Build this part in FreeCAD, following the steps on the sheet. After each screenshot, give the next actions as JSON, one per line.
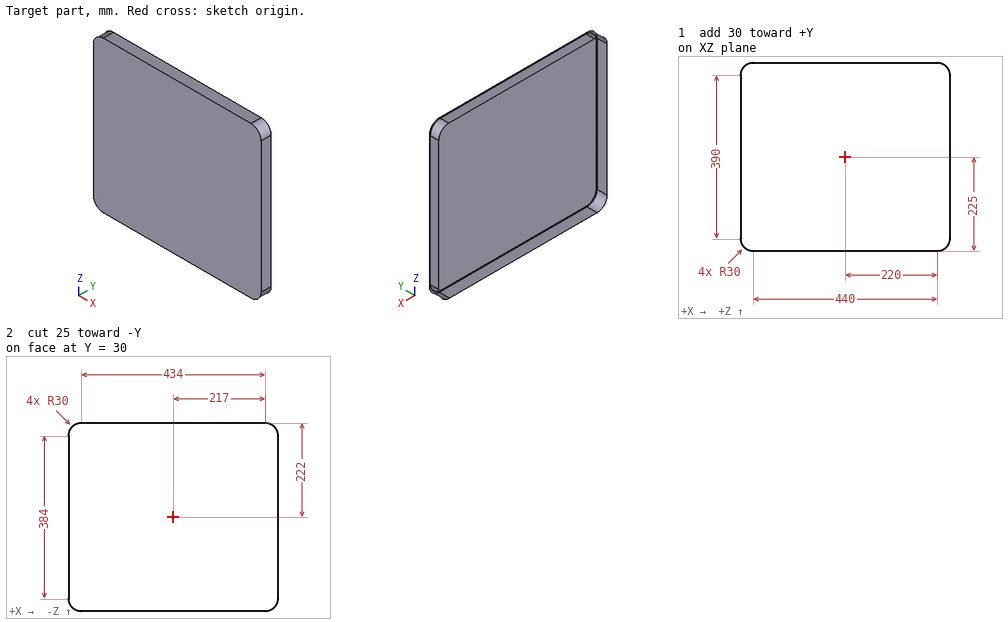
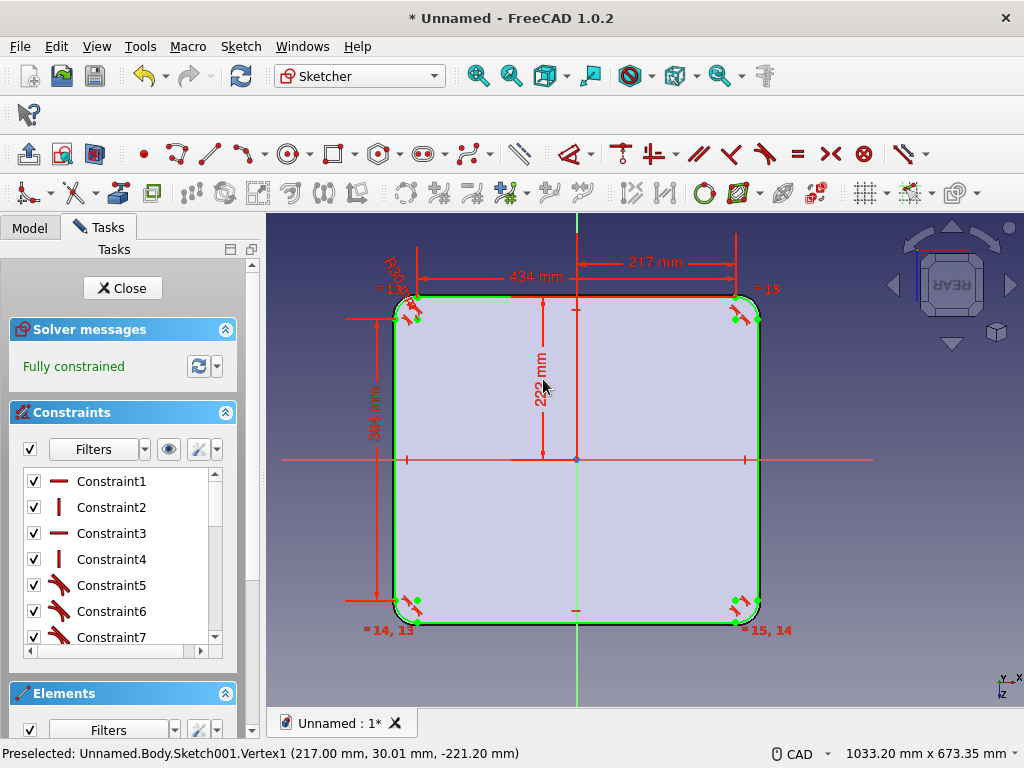
{"action": "left_click", "coordinate": [123, 288]}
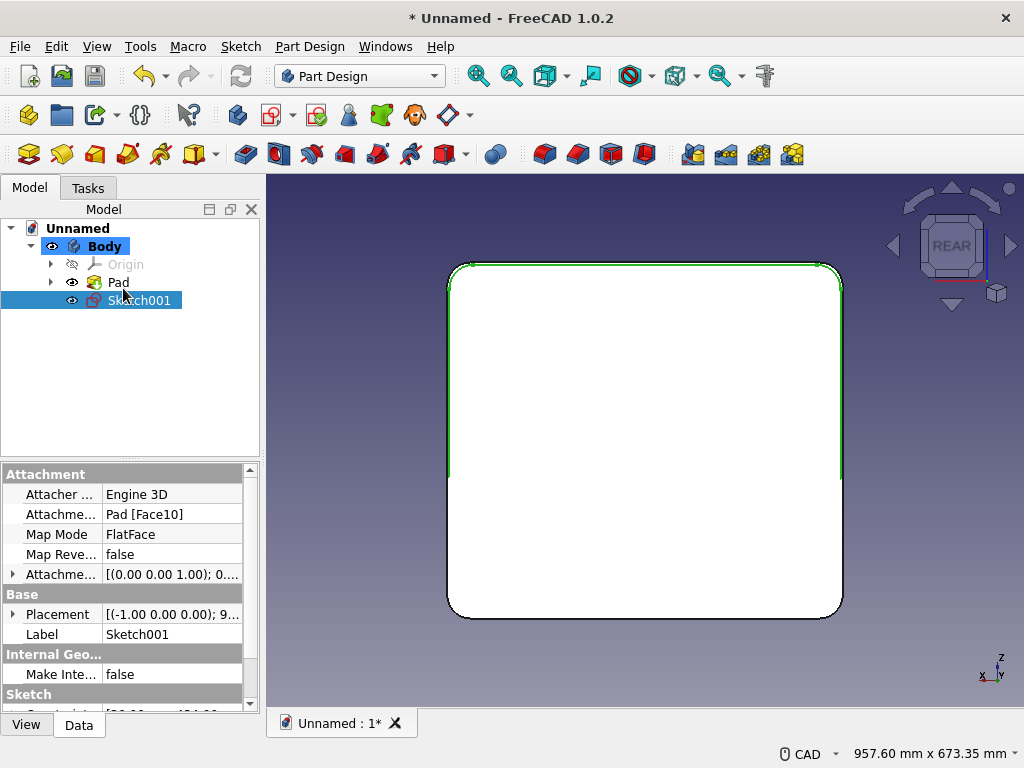
{"action": "left_click", "coordinate": [246, 154]}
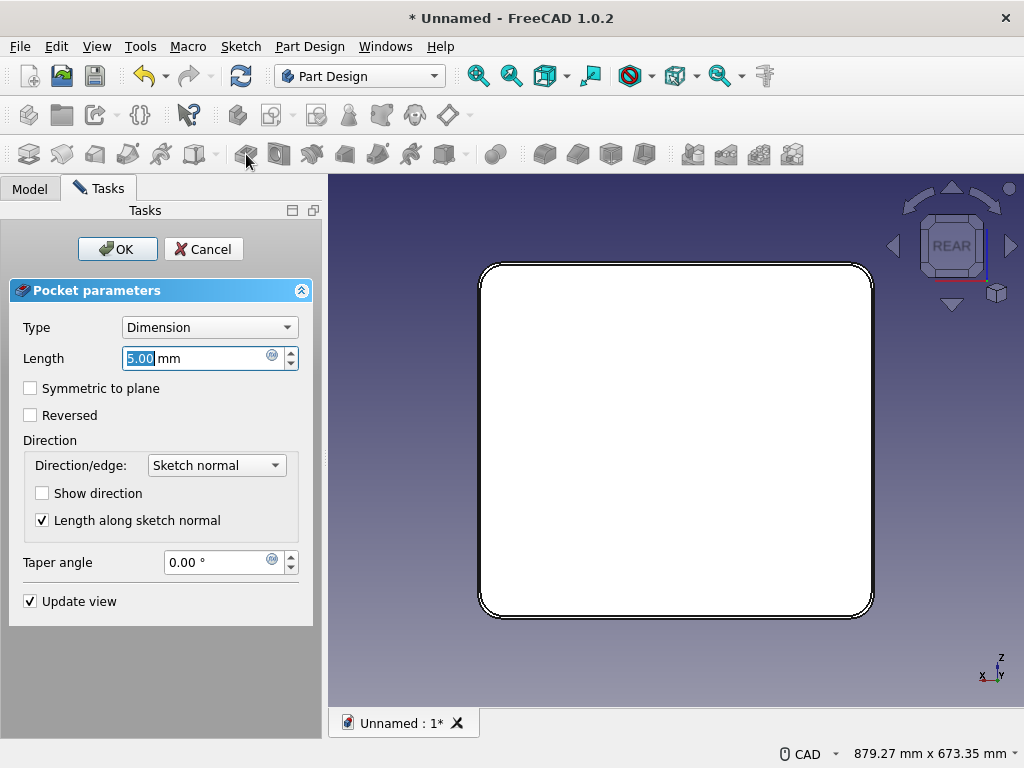
{"action": "type", "text": "25"}
{"action": "key", "text": "Tab"}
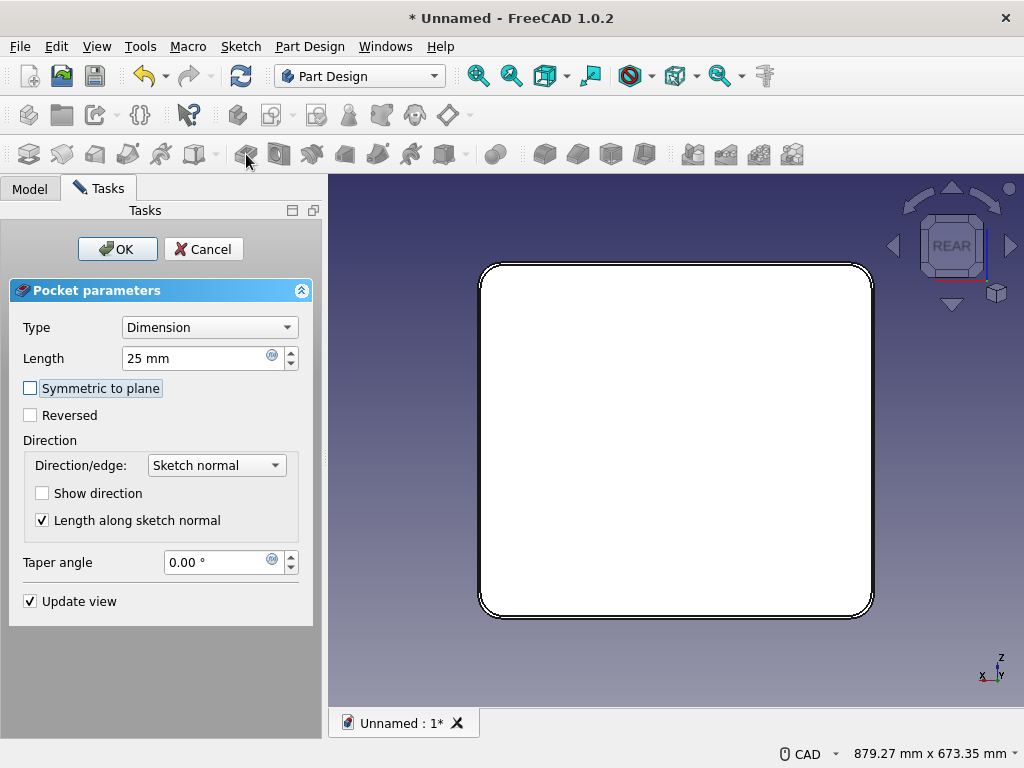
{"action": "left_click", "coordinate": [118, 249]}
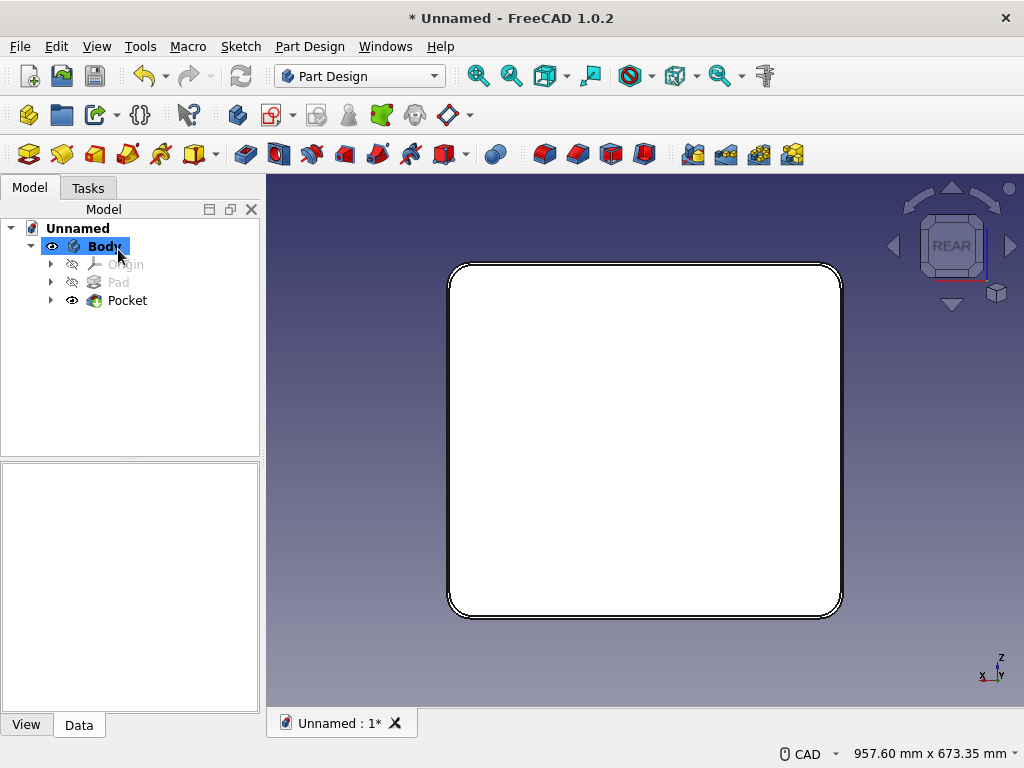
{"action": "key", "text": "0"}